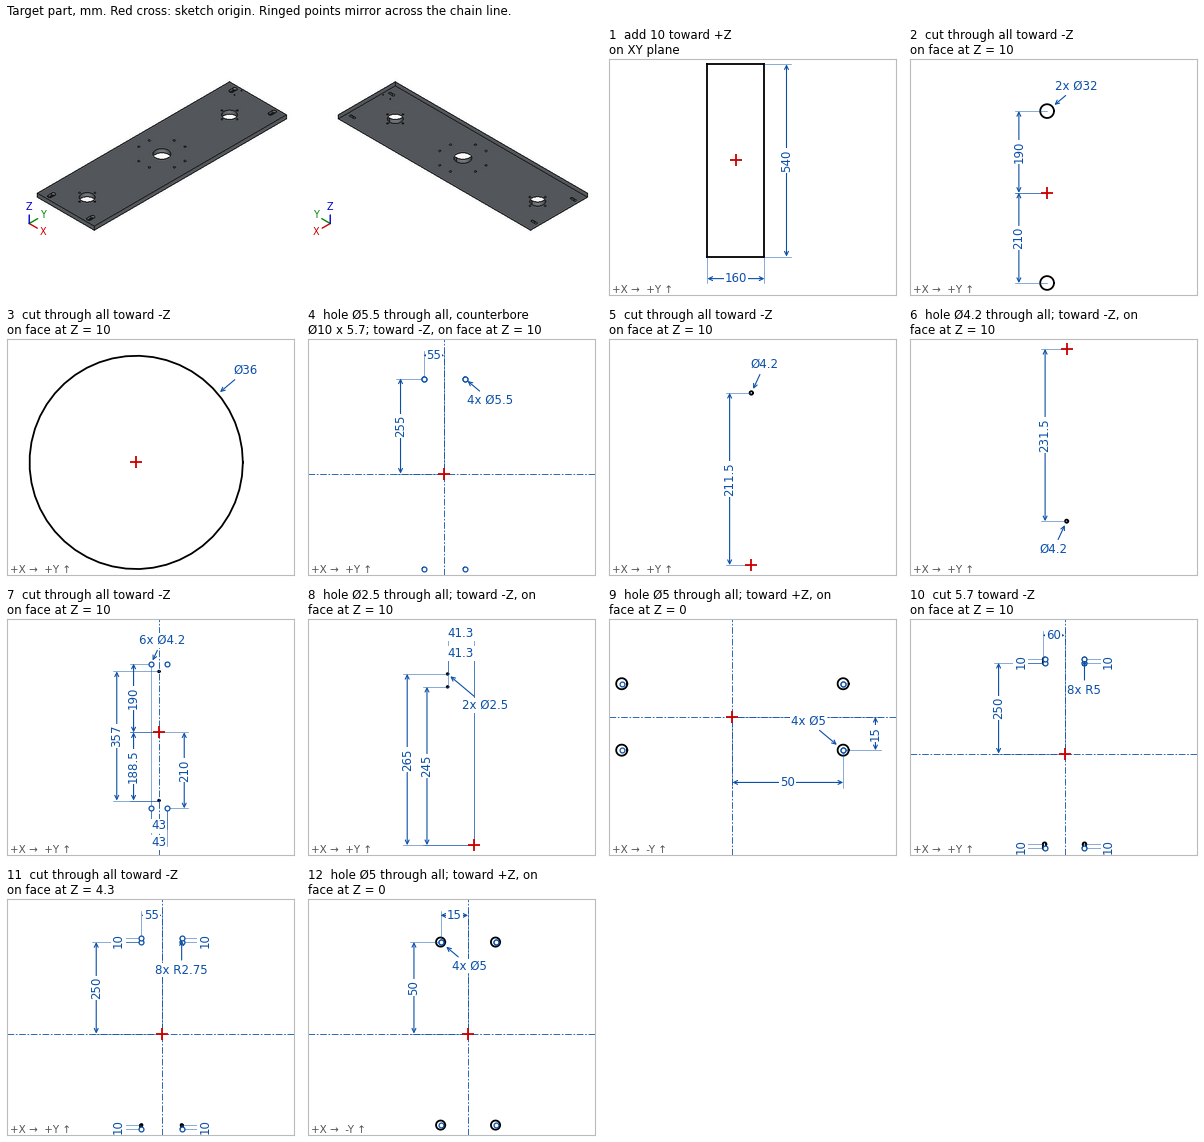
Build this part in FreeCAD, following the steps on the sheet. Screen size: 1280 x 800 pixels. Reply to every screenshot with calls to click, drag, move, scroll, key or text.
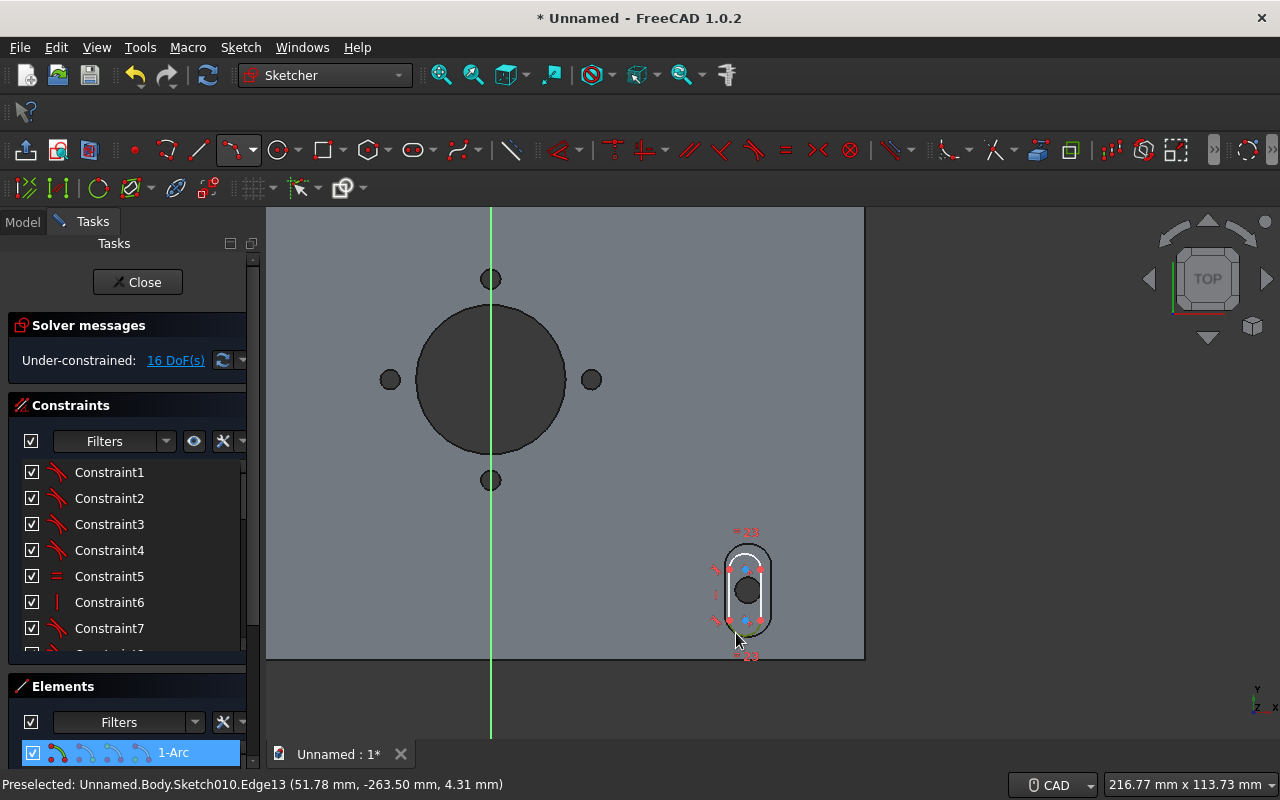
key(e)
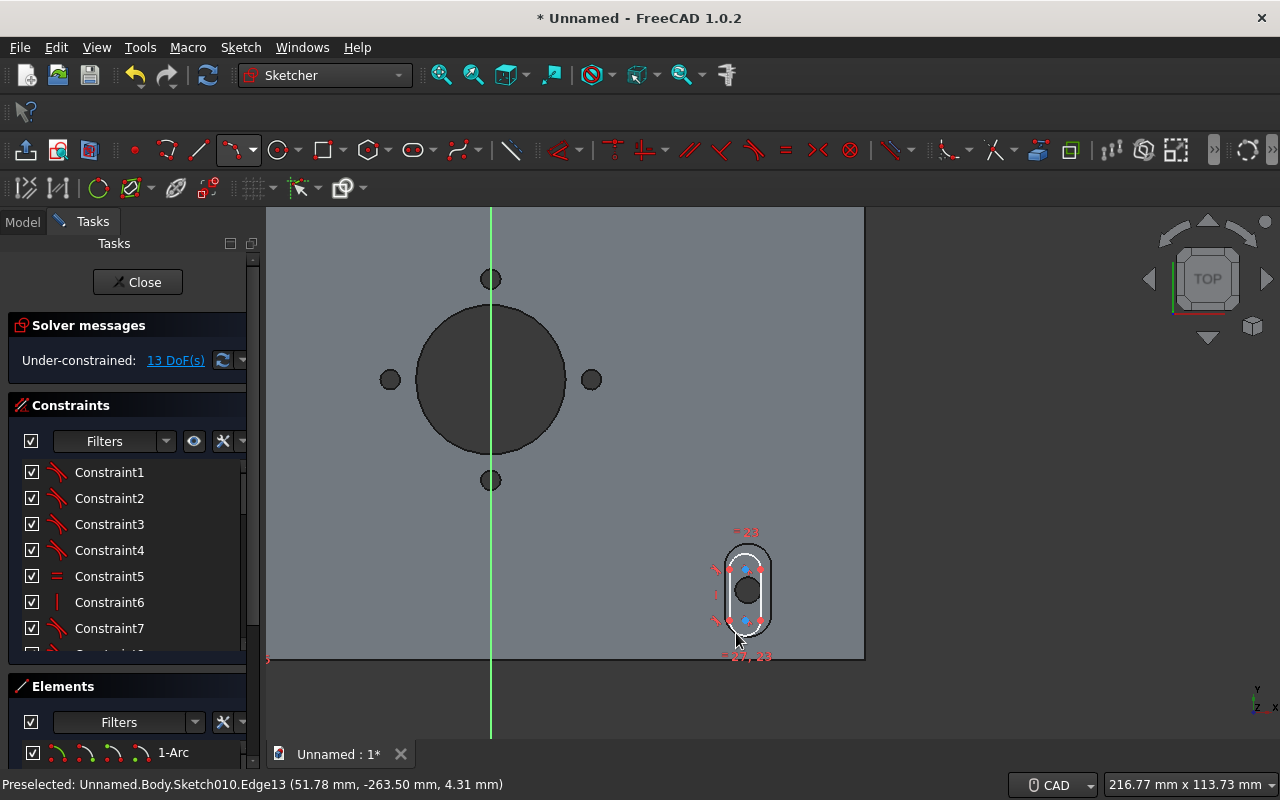
scroll(738, 641, down, 10)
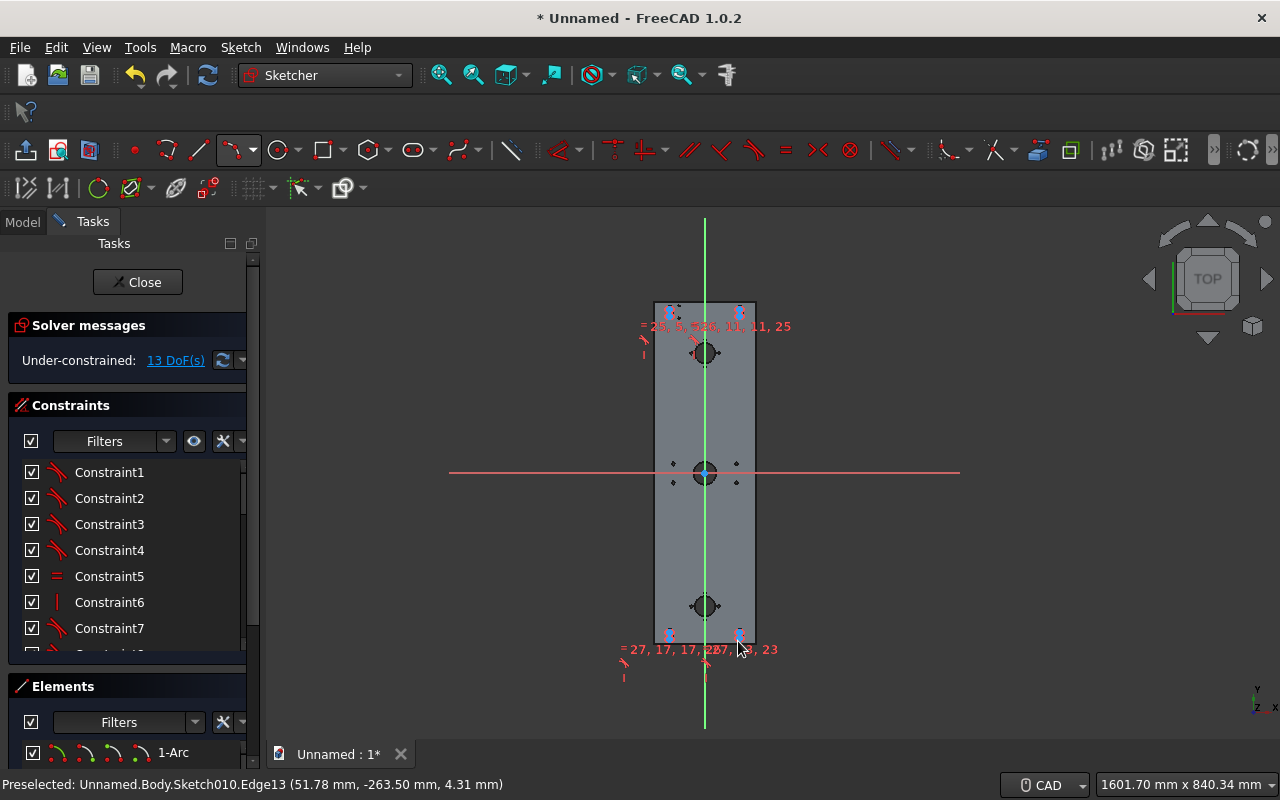
scroll(670, 316, up, 9)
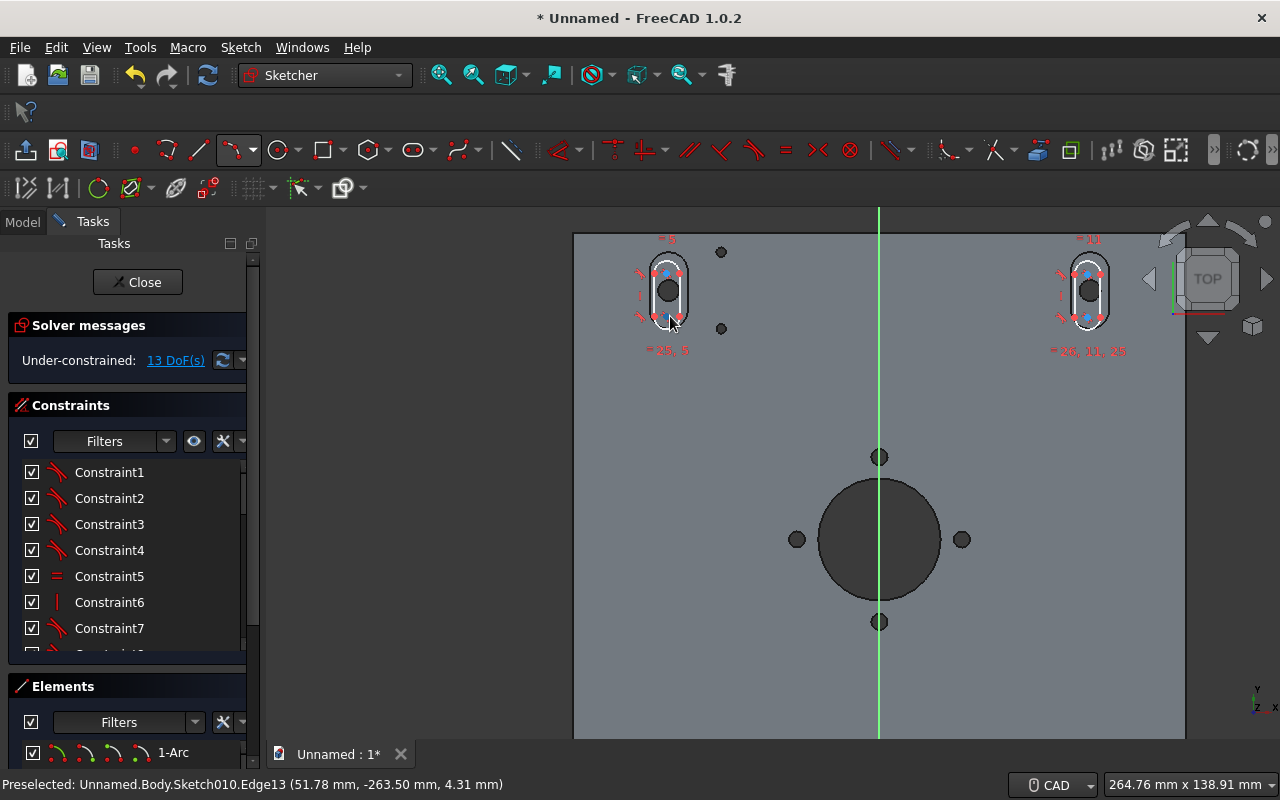
click(667, 317)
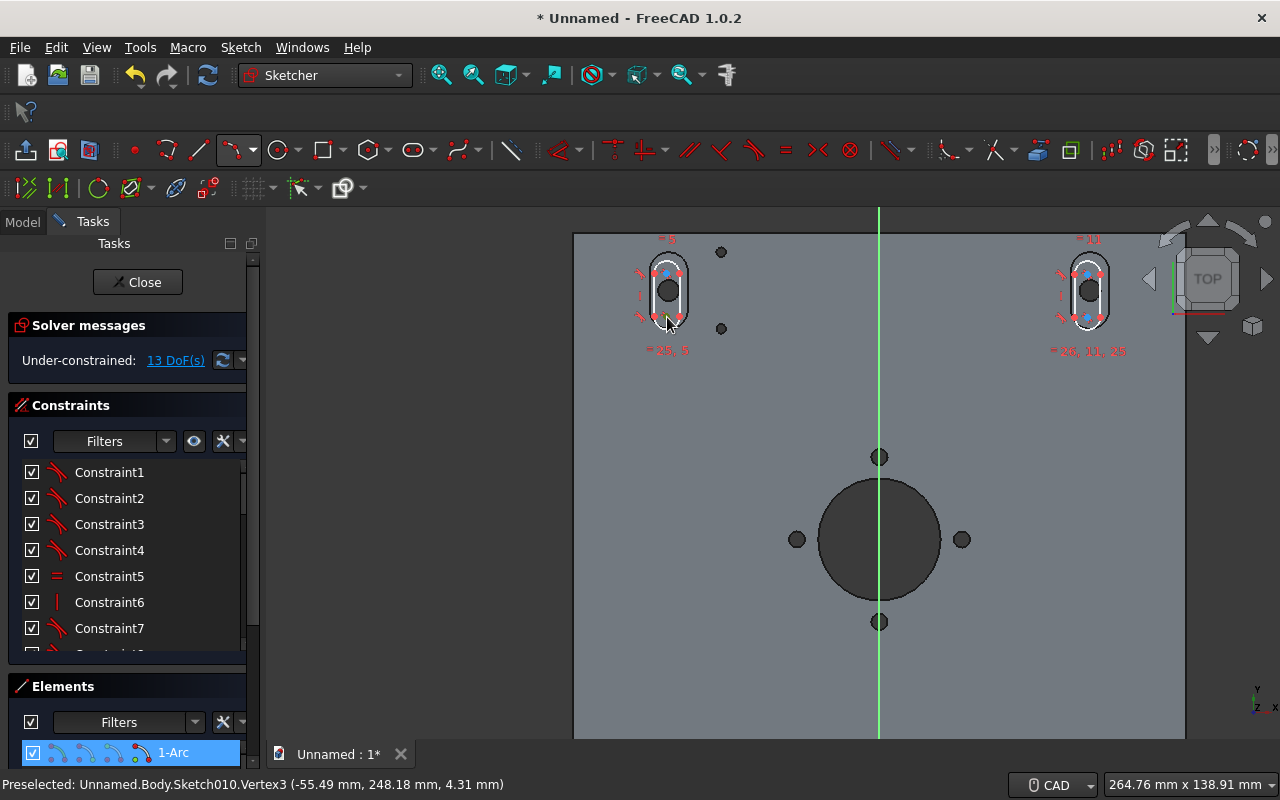
click(1088, 317)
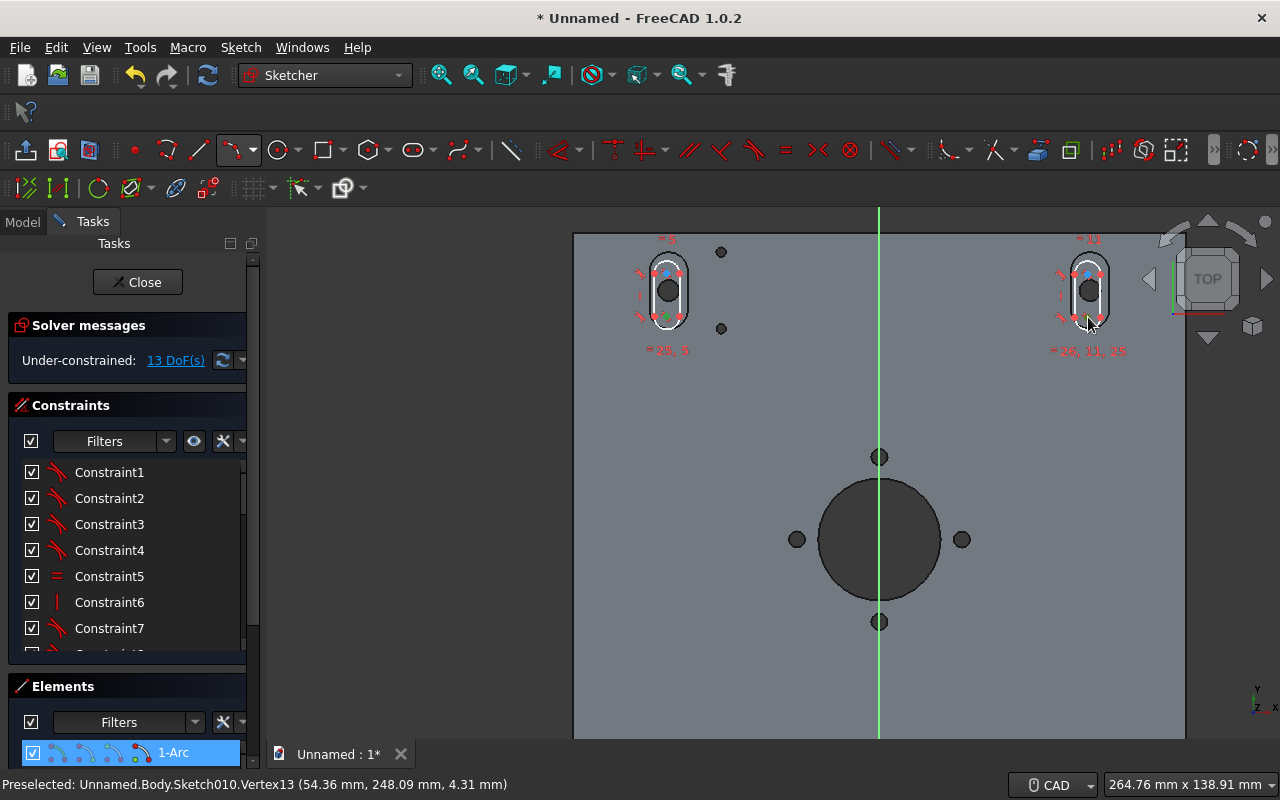
click(879, 677)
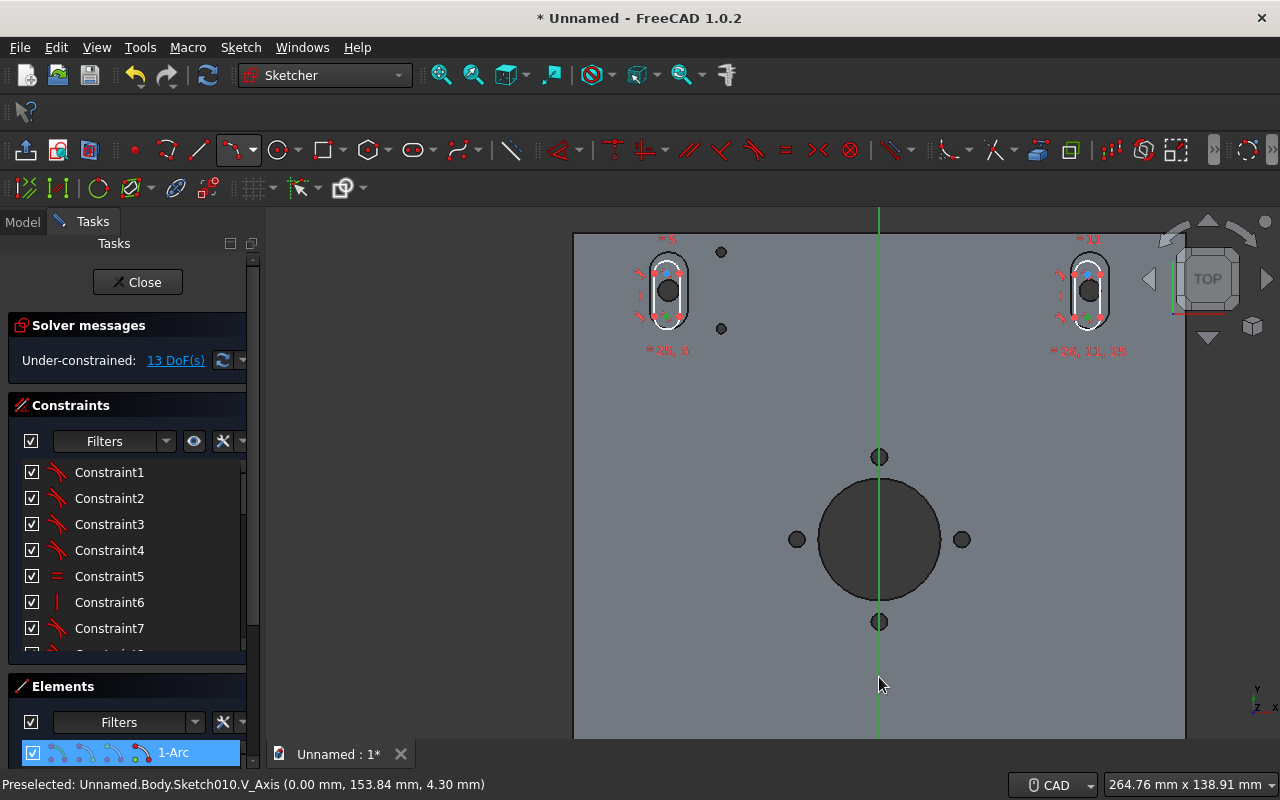
click(818, 150)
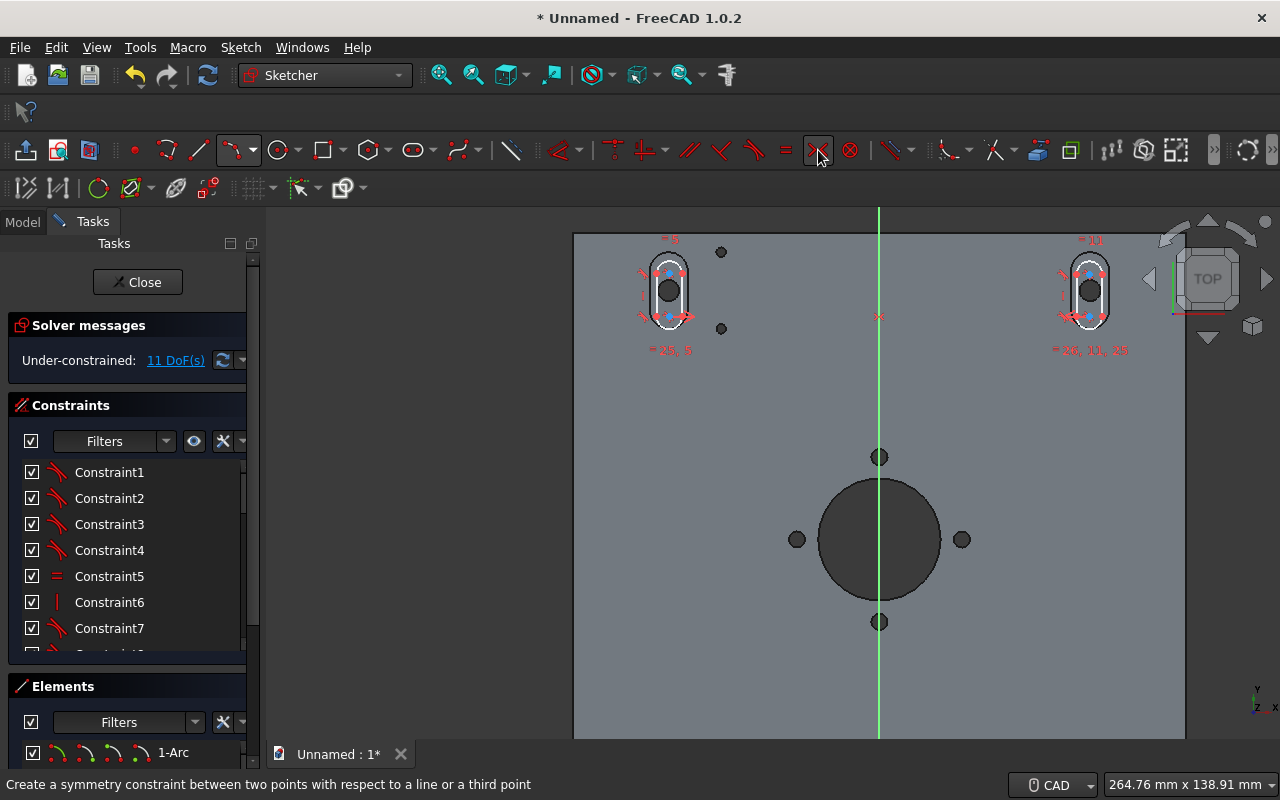
click(669, 274)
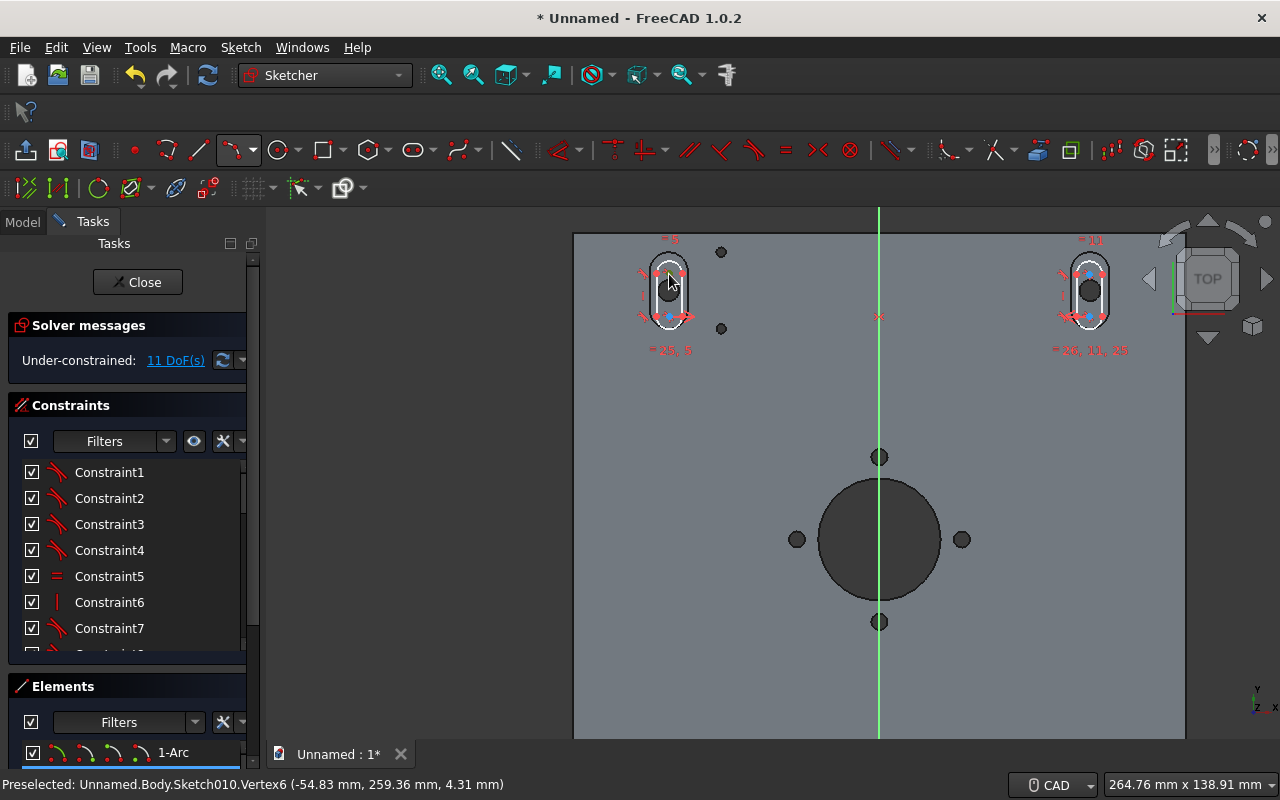
scroll(670, 316, down, 9)